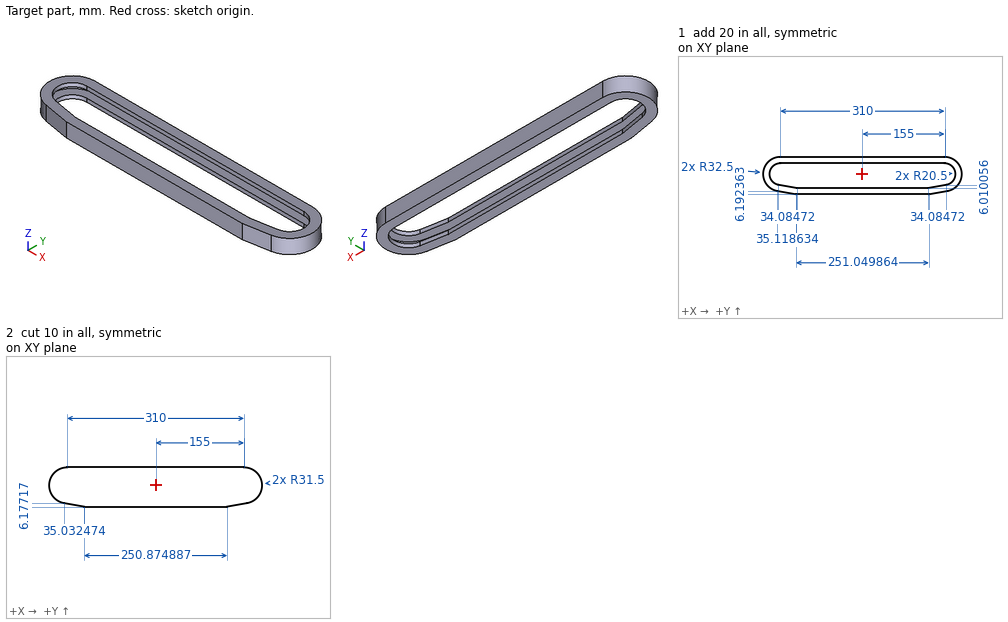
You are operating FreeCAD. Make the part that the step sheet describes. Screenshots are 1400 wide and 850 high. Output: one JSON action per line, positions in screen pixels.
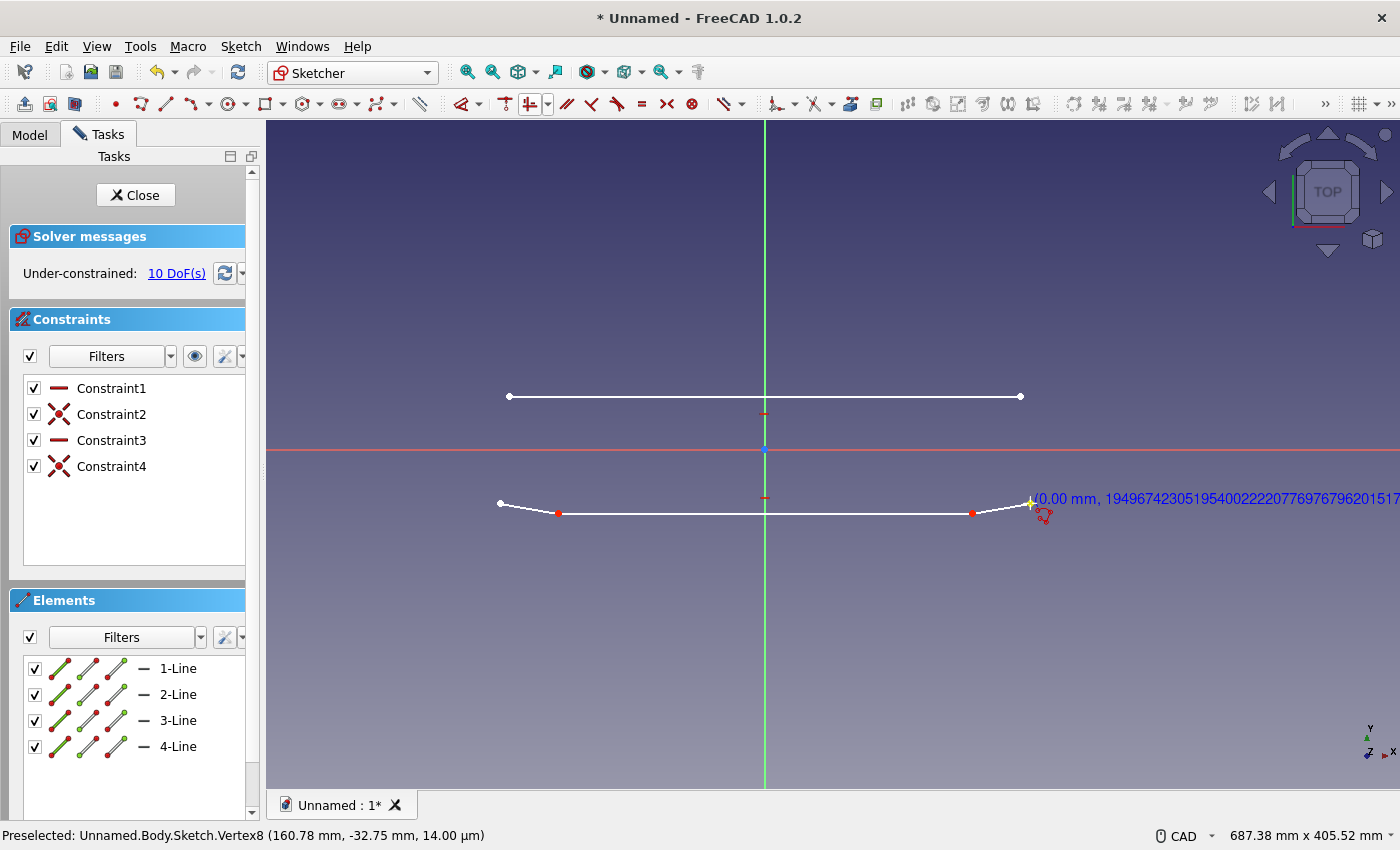
{"action": "key", "text": "g 3 a"}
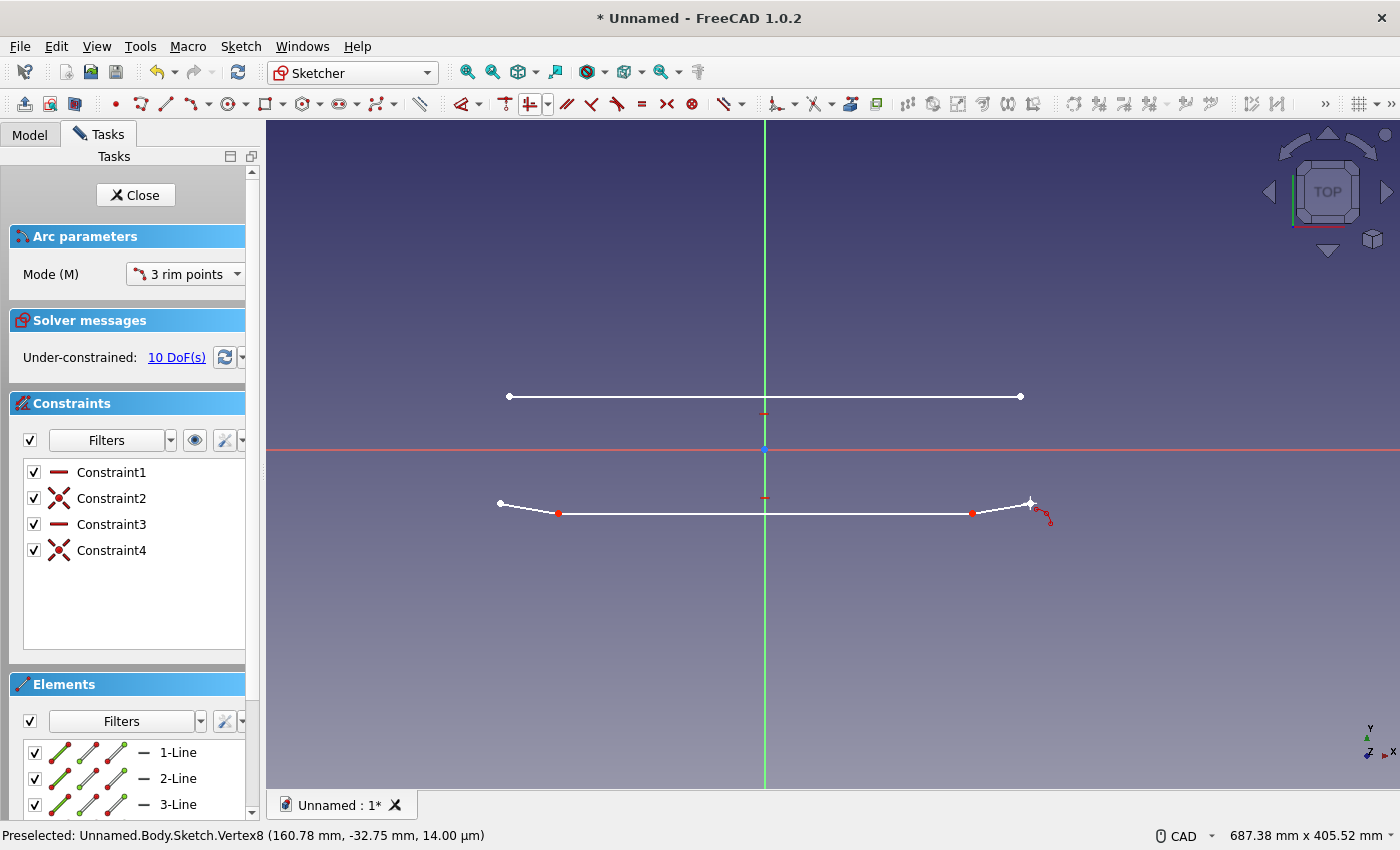
{"action": "left_click", "coordinate": [509, 397]}
{"action": "left_click", "coordinate": [500, 504]}
{"action": "left_click", "coordinate": [459, 430]}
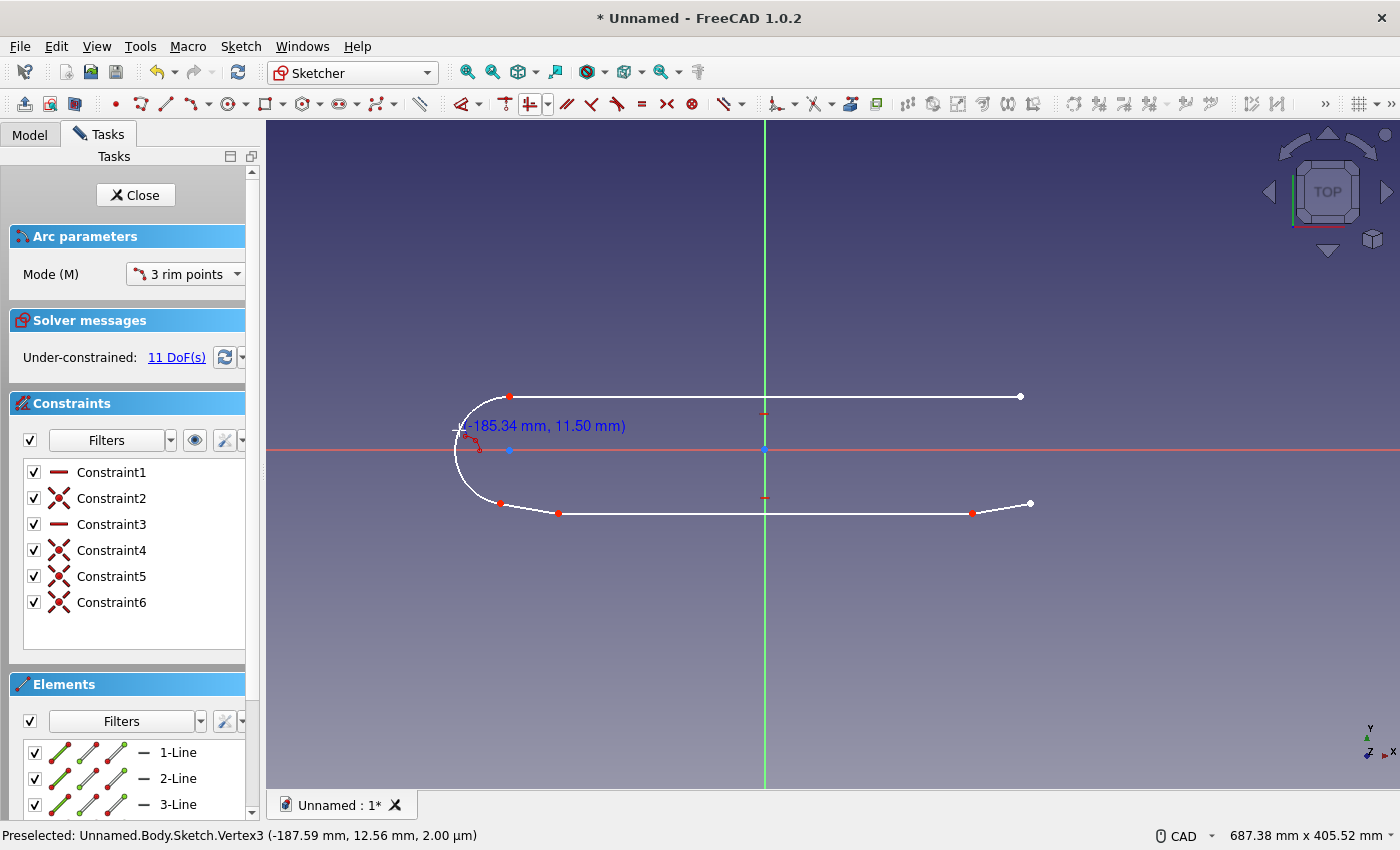
{"action": "left_click", "coordinate": [1030, 504]}
{"action": "left_click", "coordinate": [1020, 397]}
{"action": "left_click", "coordinate": [1070, 430]}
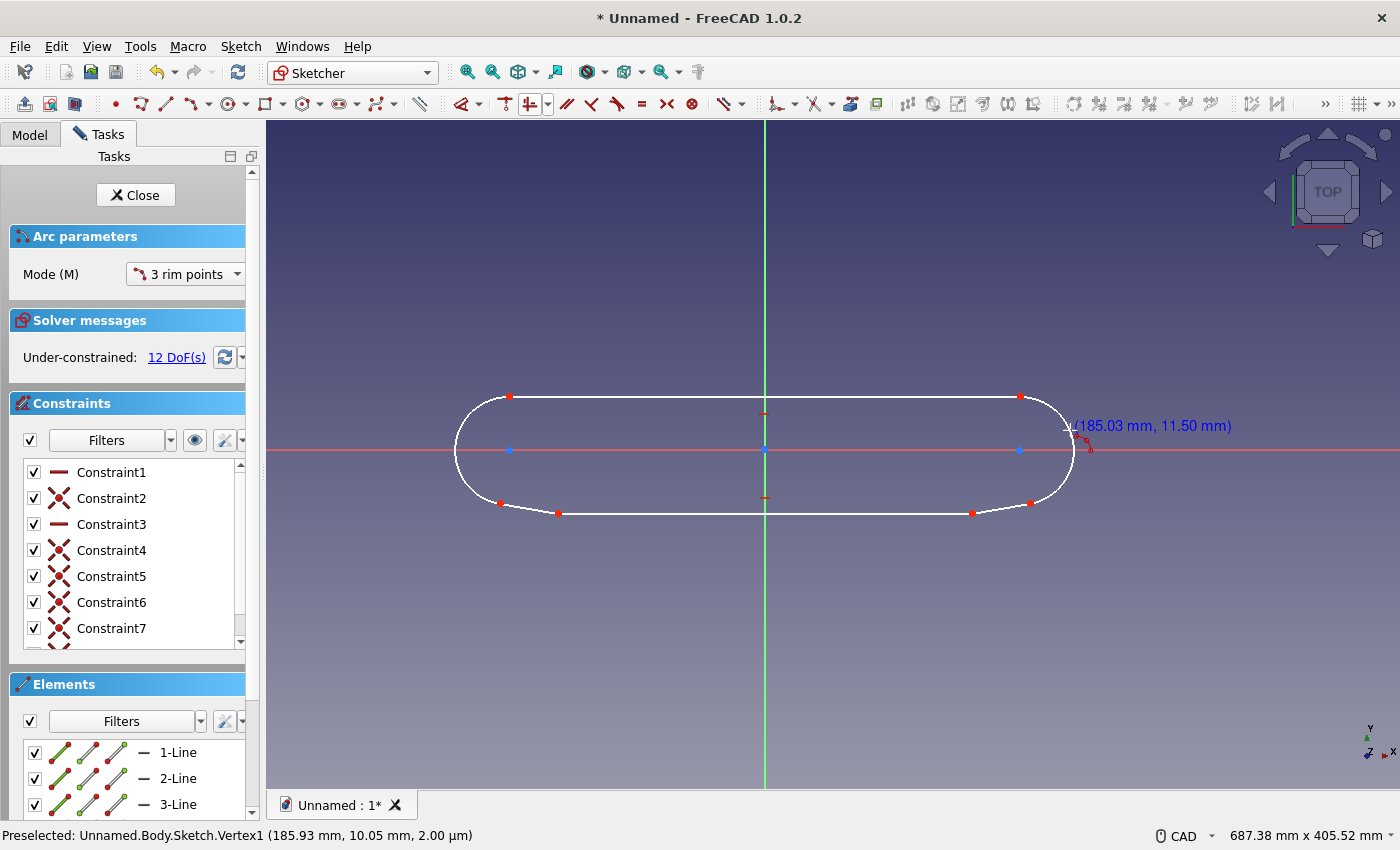
{"action": "key", "text": "g l"}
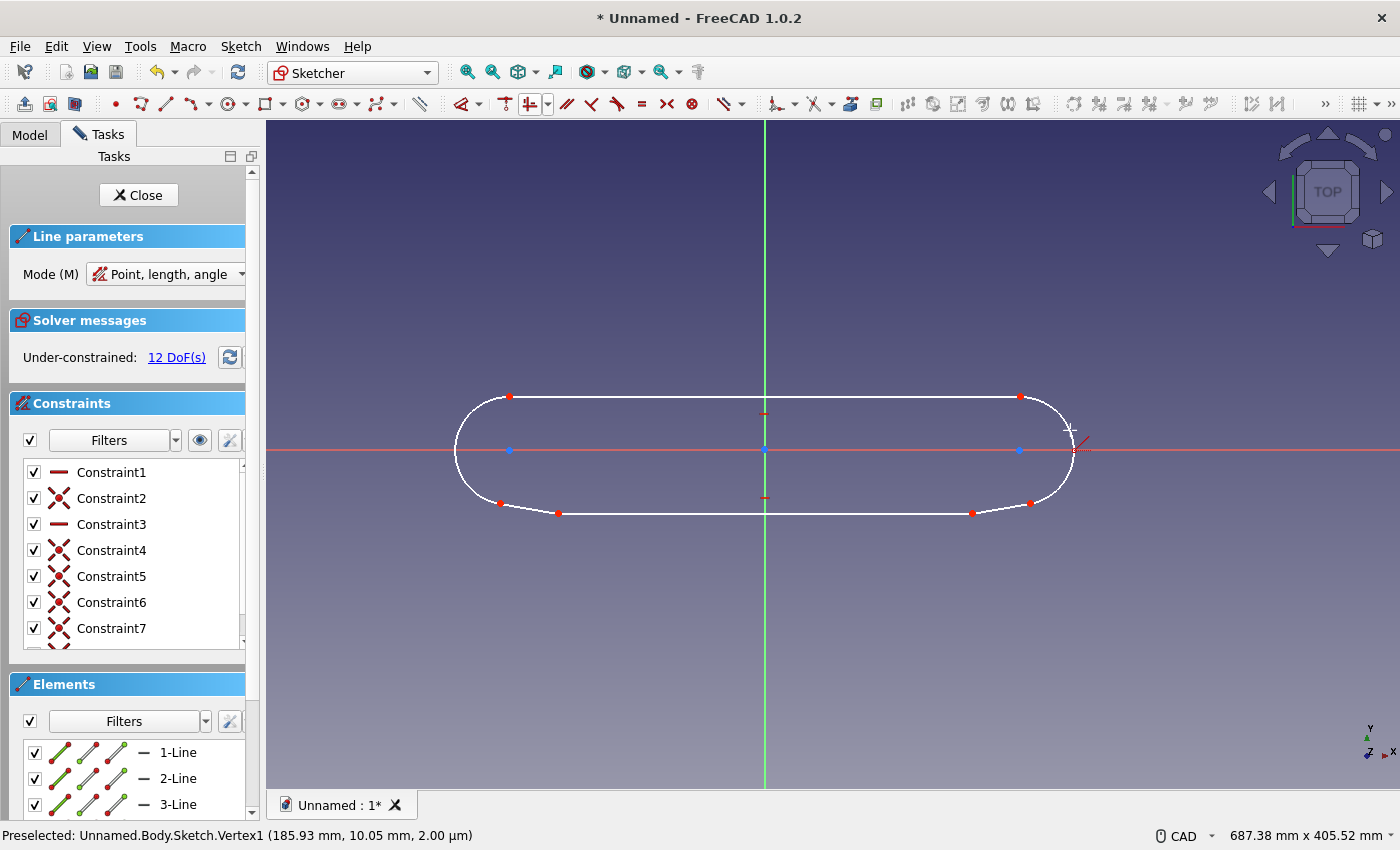
{"action": "left_click", "coordinate": [509, 416]}
{"action": "left_click", "coordinate": [1020, 416]}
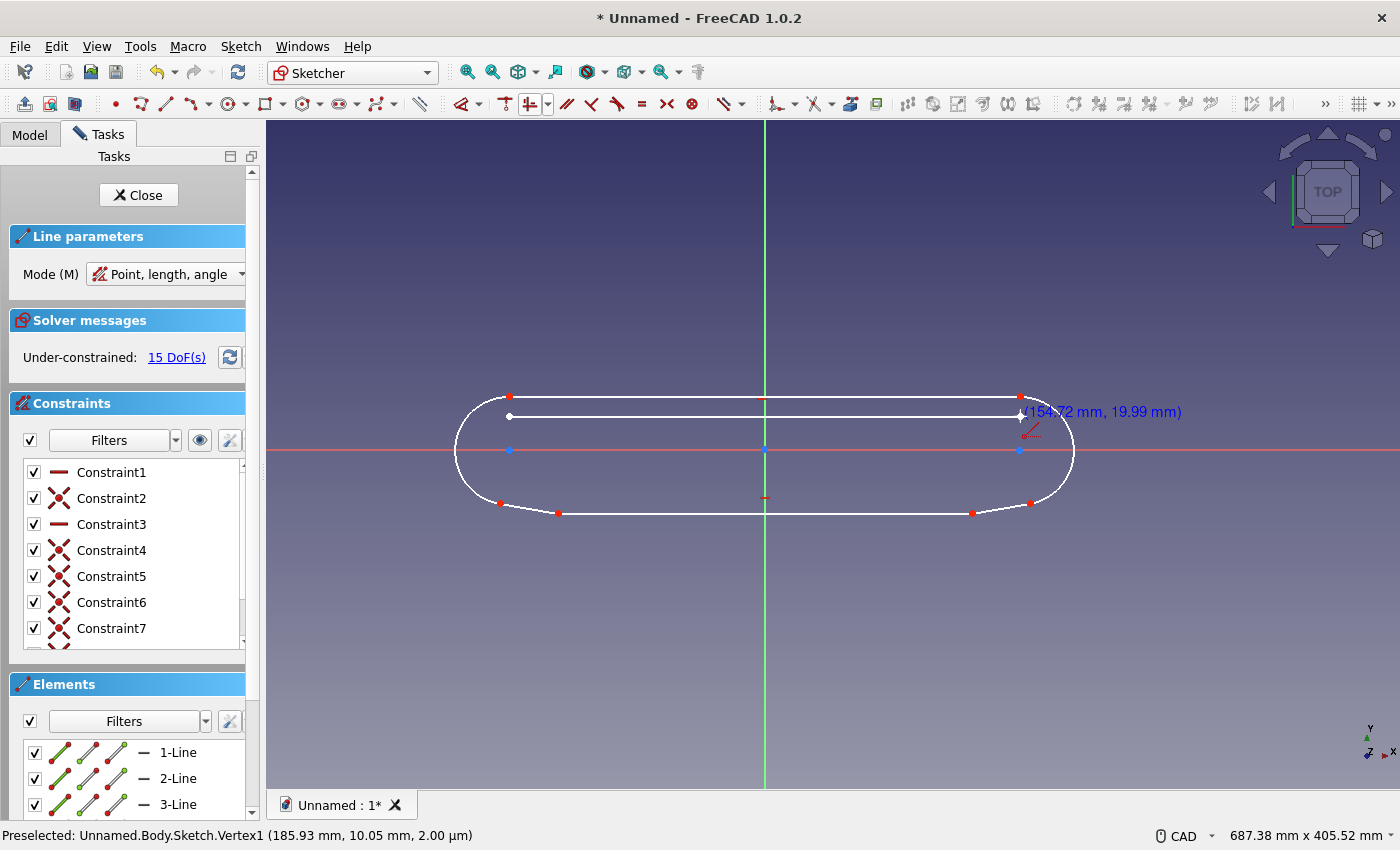
{"action": "left_click", "coordinate": [141, 104]}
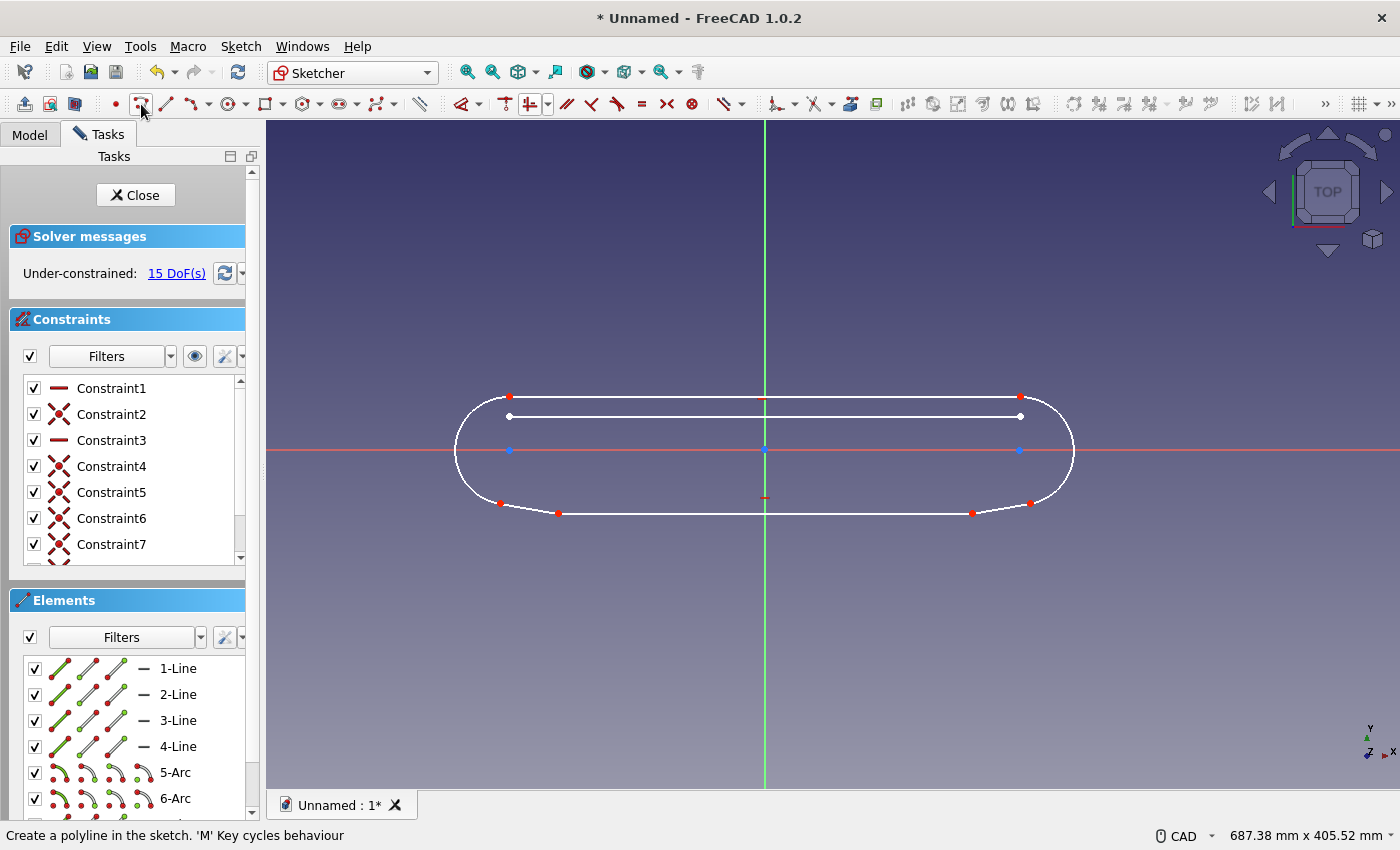
{"action": "left_click", "coordinate": [1026, 483]}
{"action": "left_click", "coordinate": [970, 493]}
{"action": "left_click", "coordinate": [559, 493]}
{"action": "left_click", "coordinate": [503, 483]}
{"action": "right_click", "coordinate": [503, 483]}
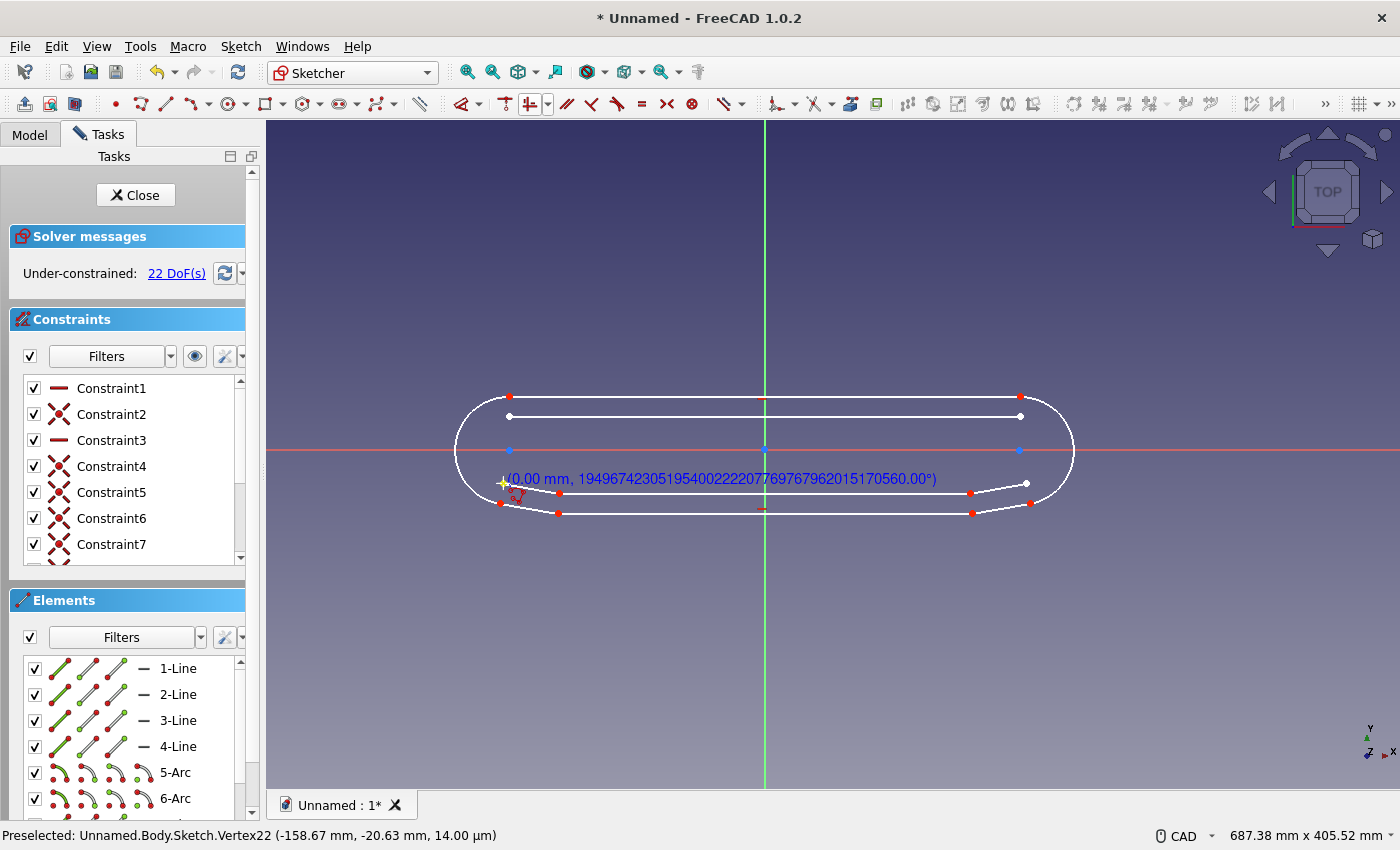
{"action": "key", "text": "g 3 a"}